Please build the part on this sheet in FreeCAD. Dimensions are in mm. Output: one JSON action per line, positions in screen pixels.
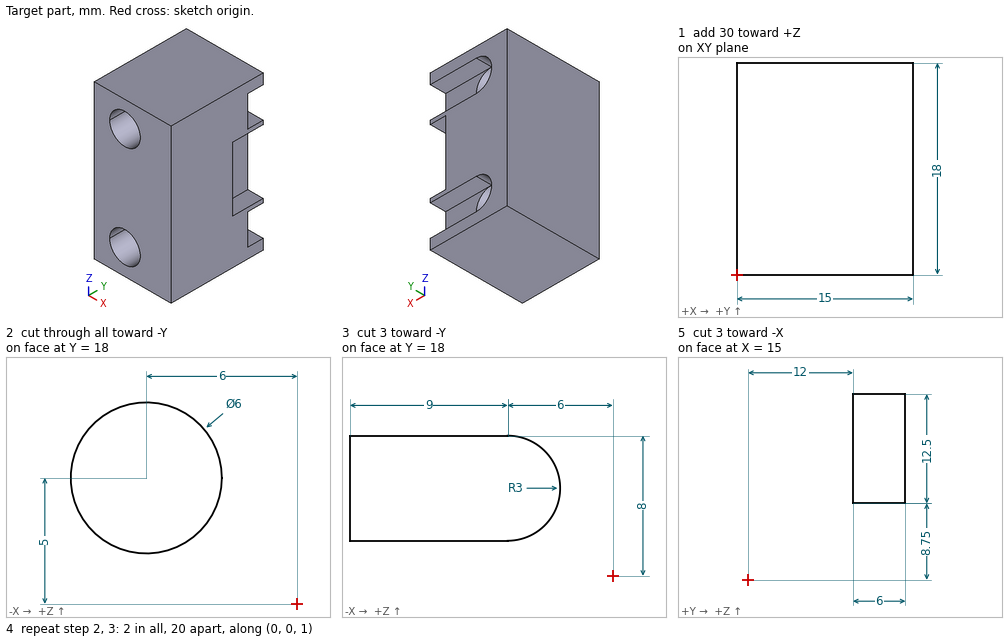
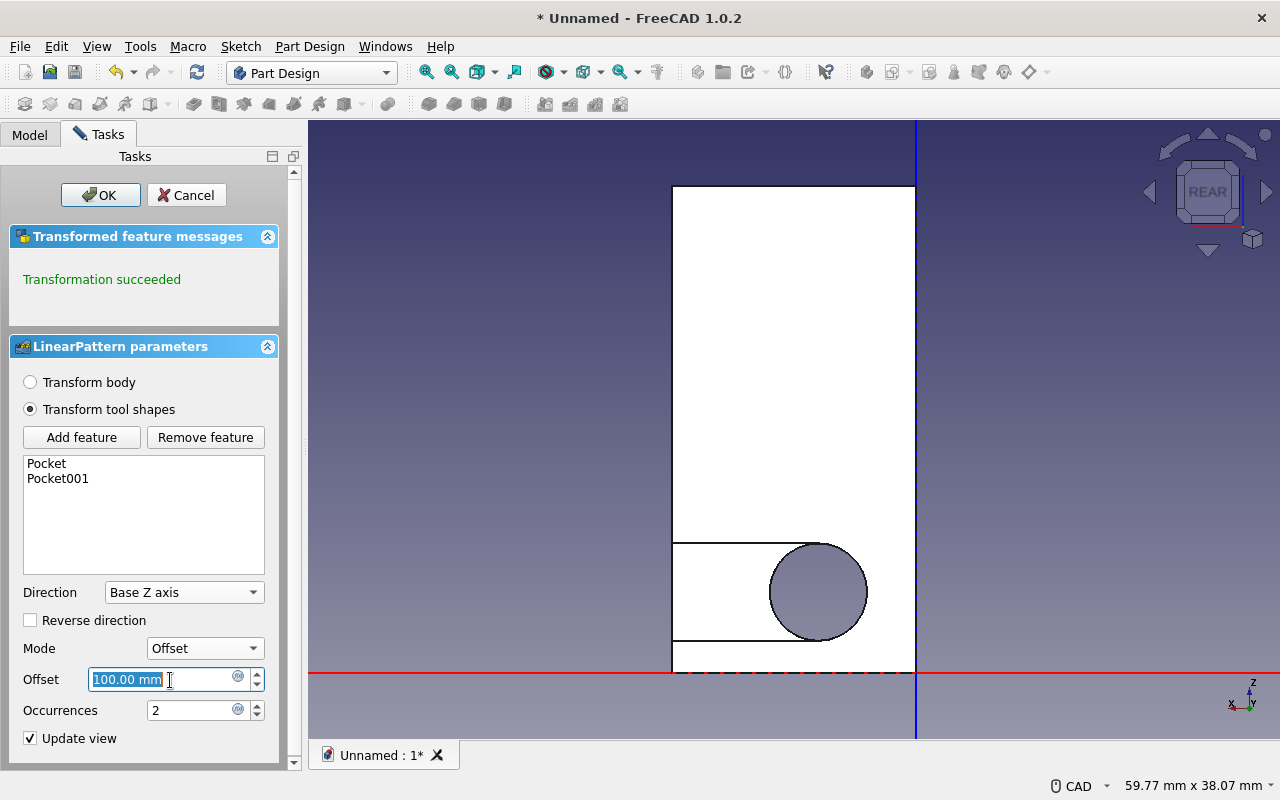
{"action": "type", "text": "20"}
{"action": "key", "text": "Tab"}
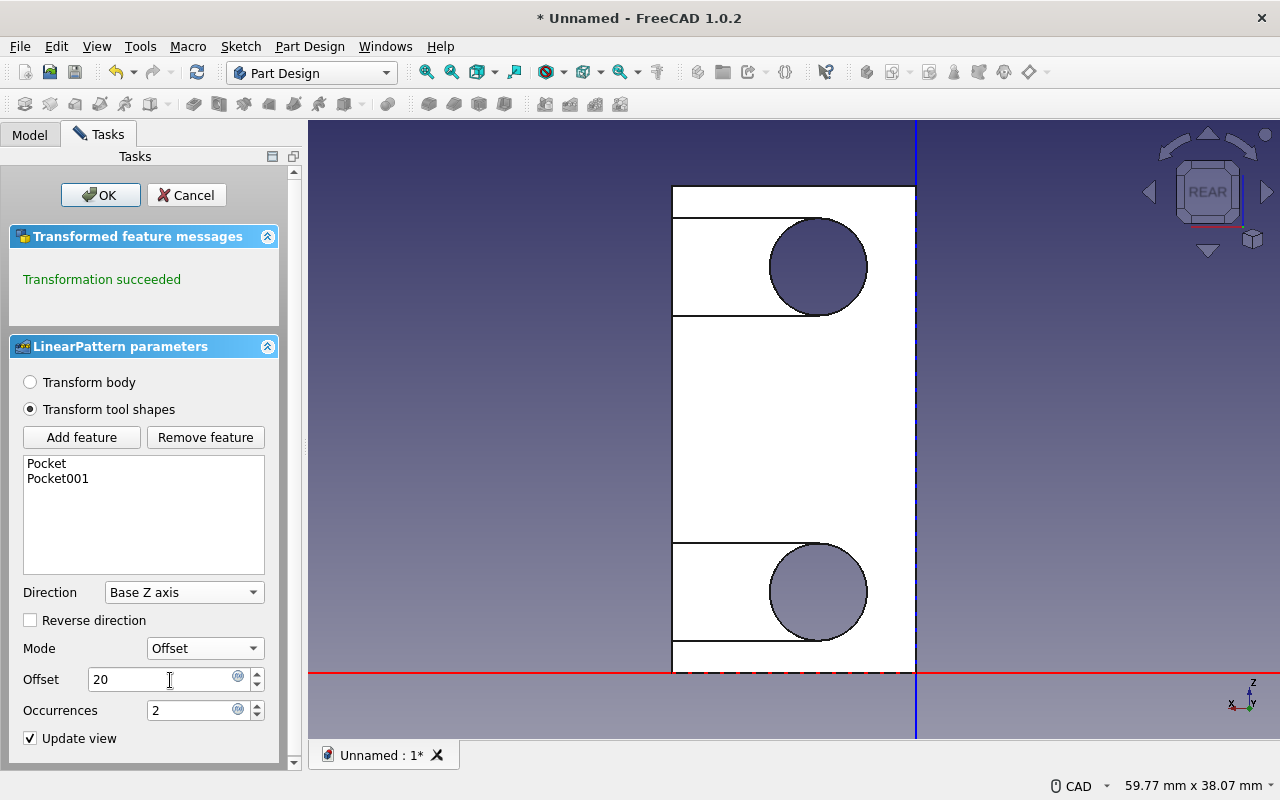
{"action": "triple_click", "coordinate": [199, 710]}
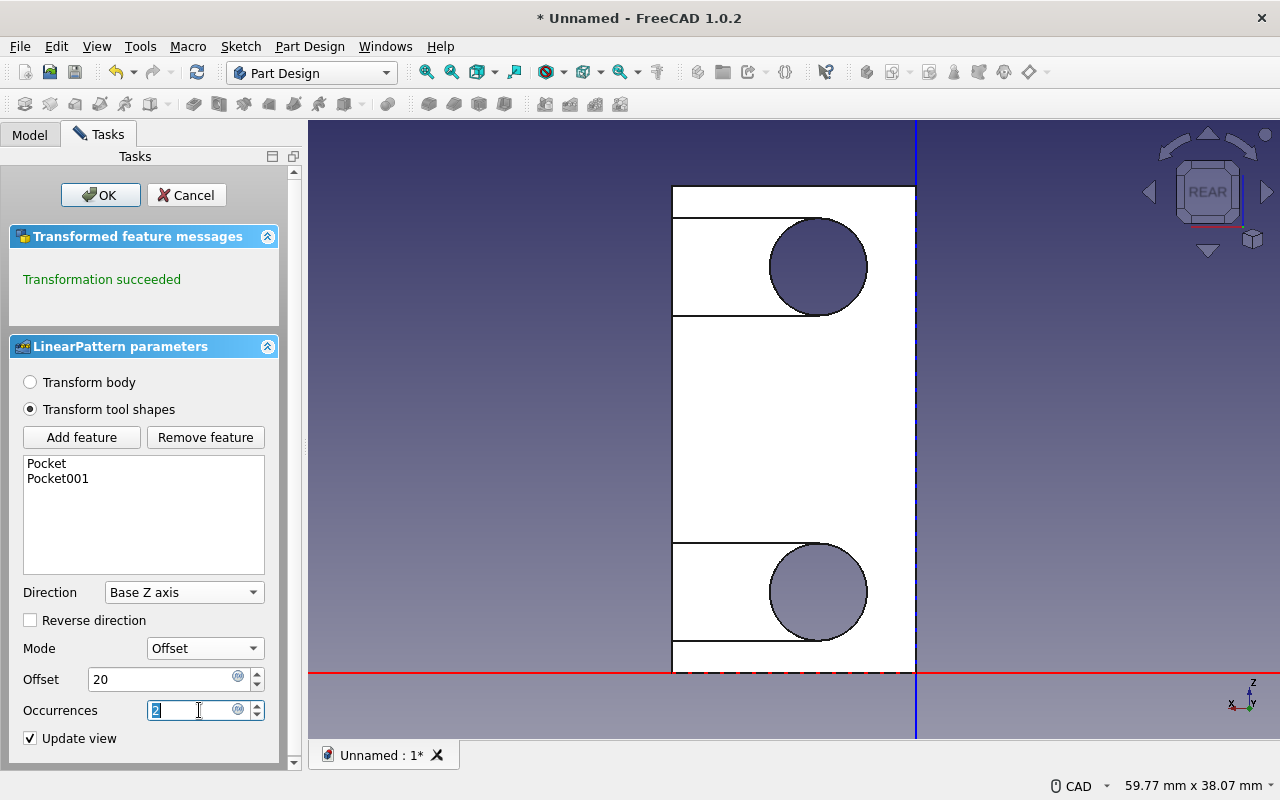
{"action": "type", "text": "2"}
{"action": "key", "text": "Tab"}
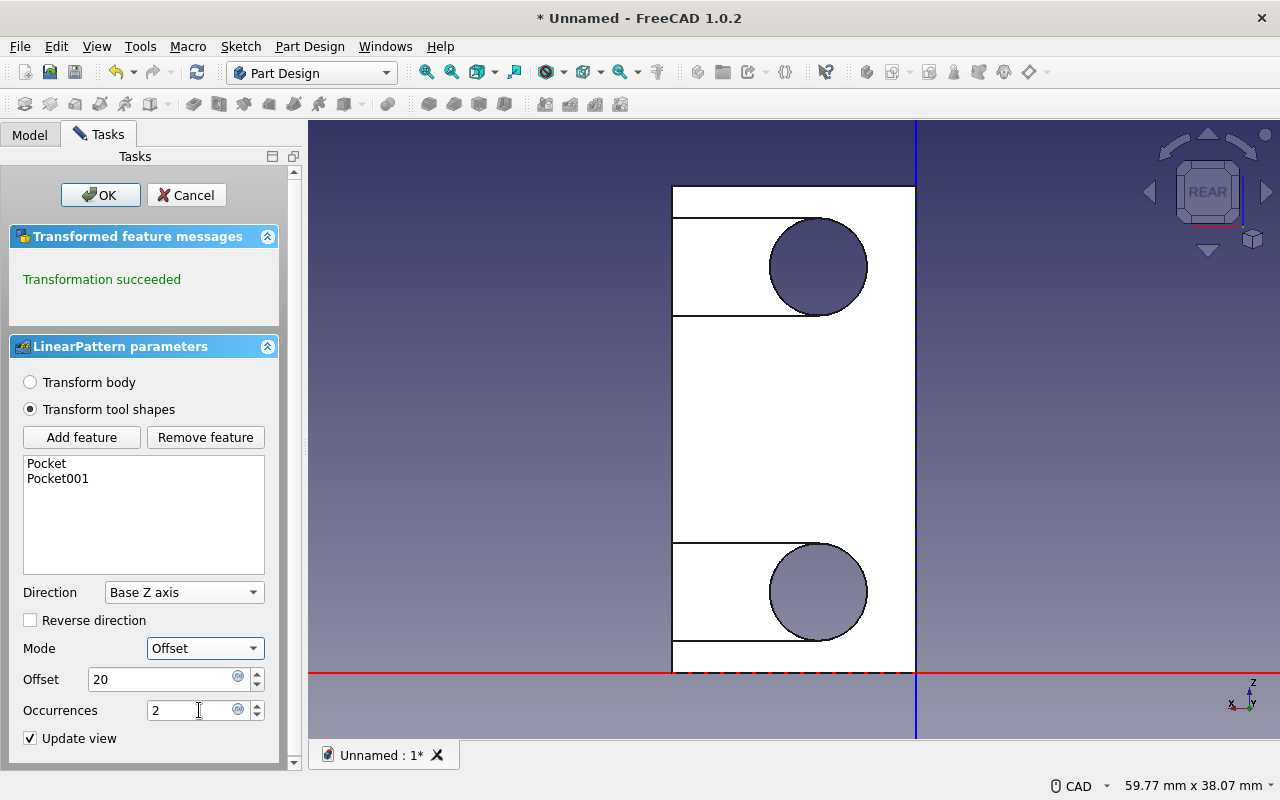
{"action": "left_click", "coordinate": [101, 195]}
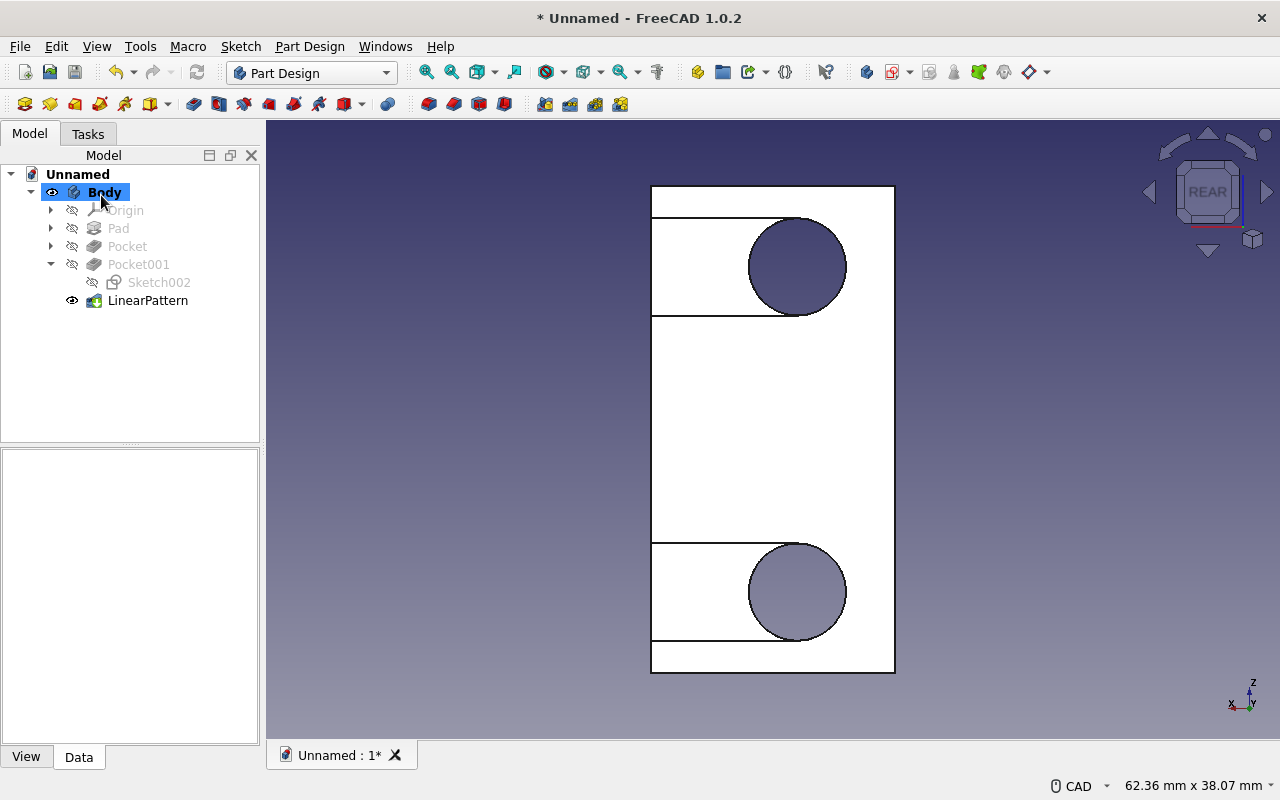
{"action": "key", "text": "0"}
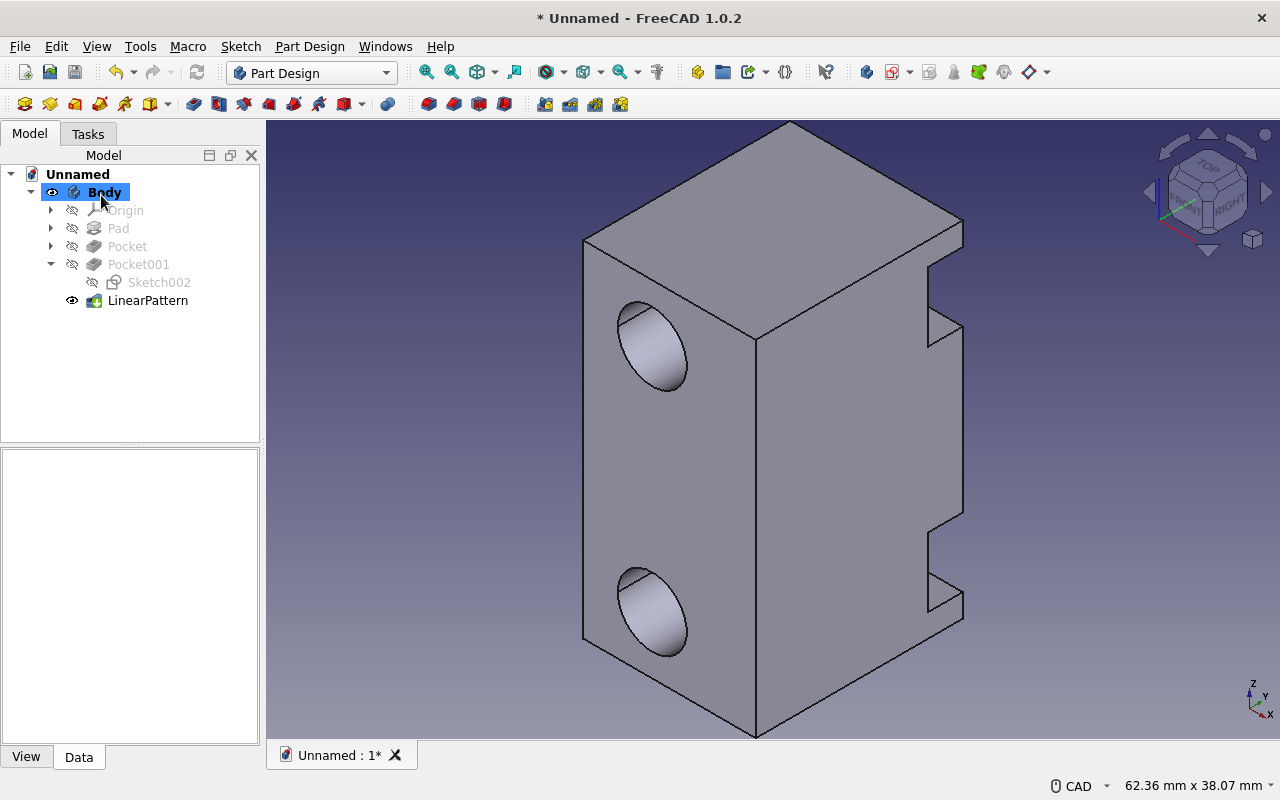
{"action": "left_click", "coordinate": [859, 478]}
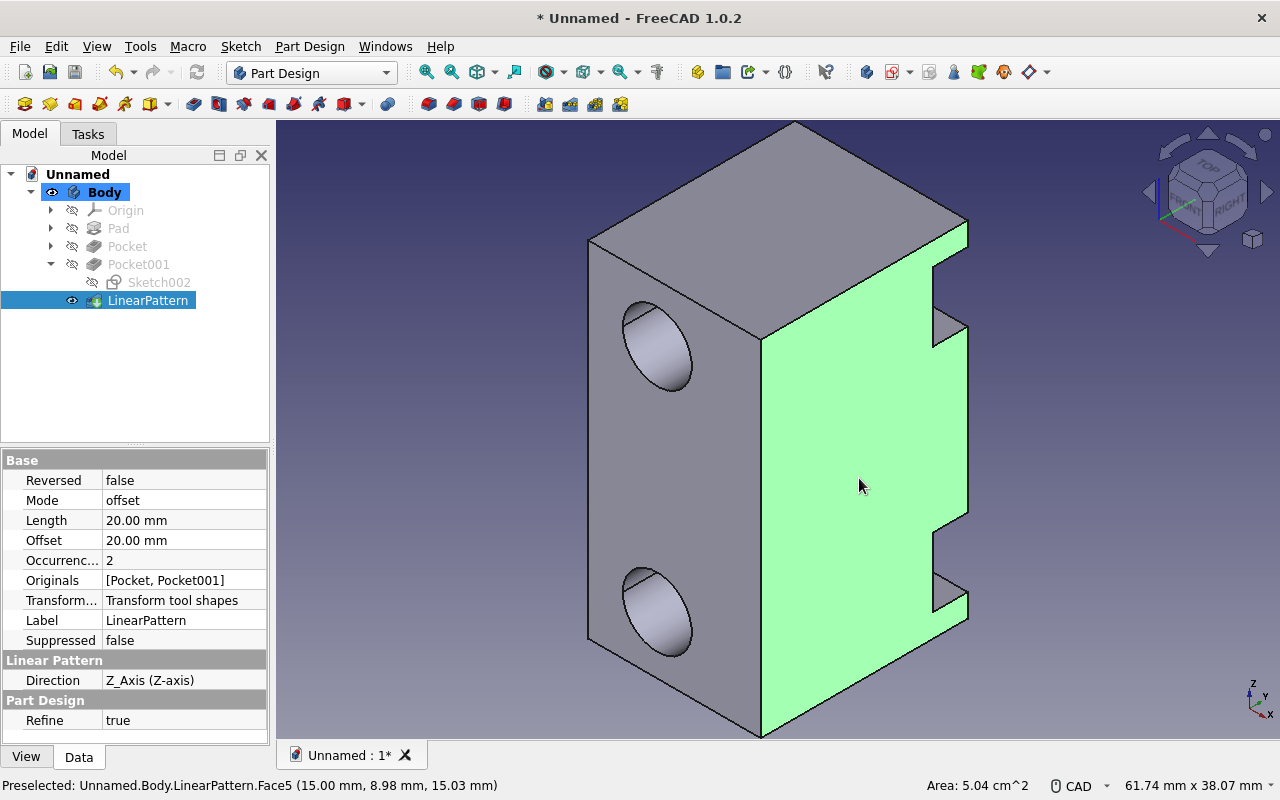
{"action": "left_click", "coordinate": [892, 72]}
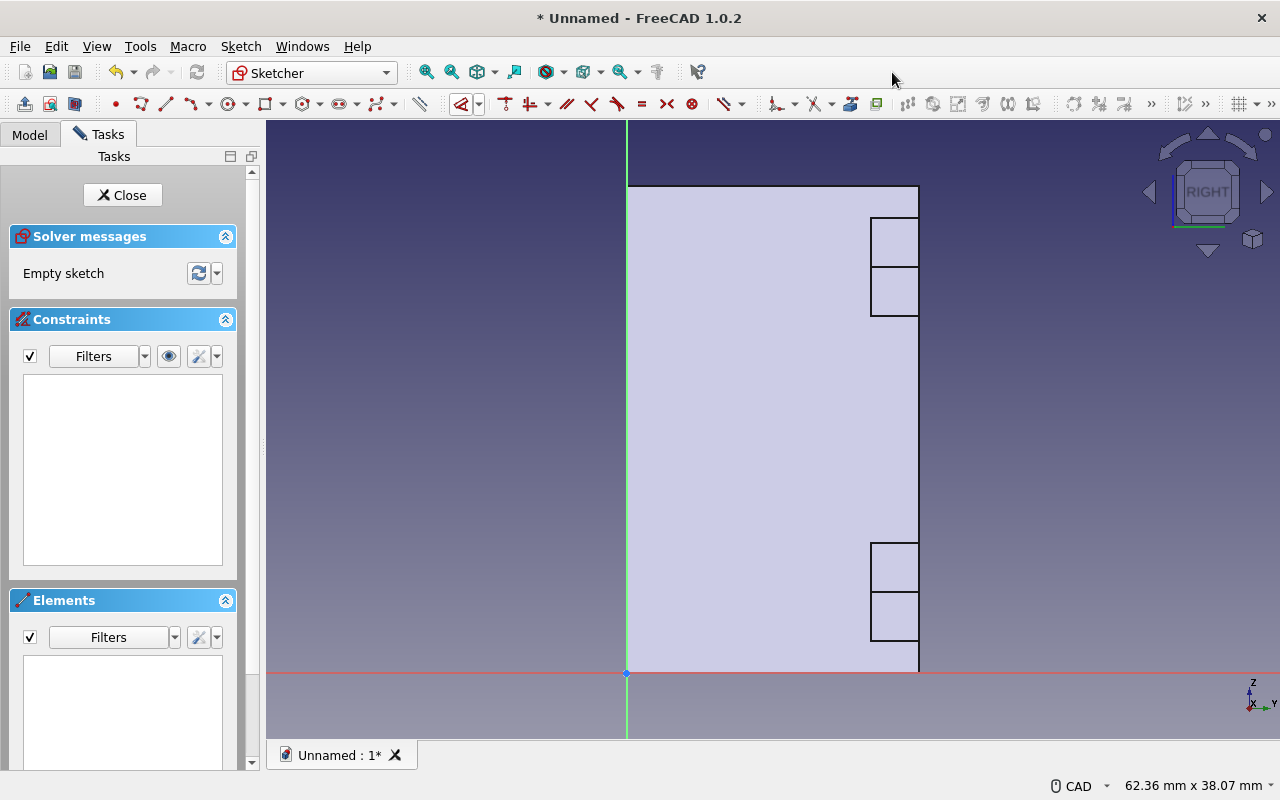
{"action": "left_click", "coordinate": [264, 104]}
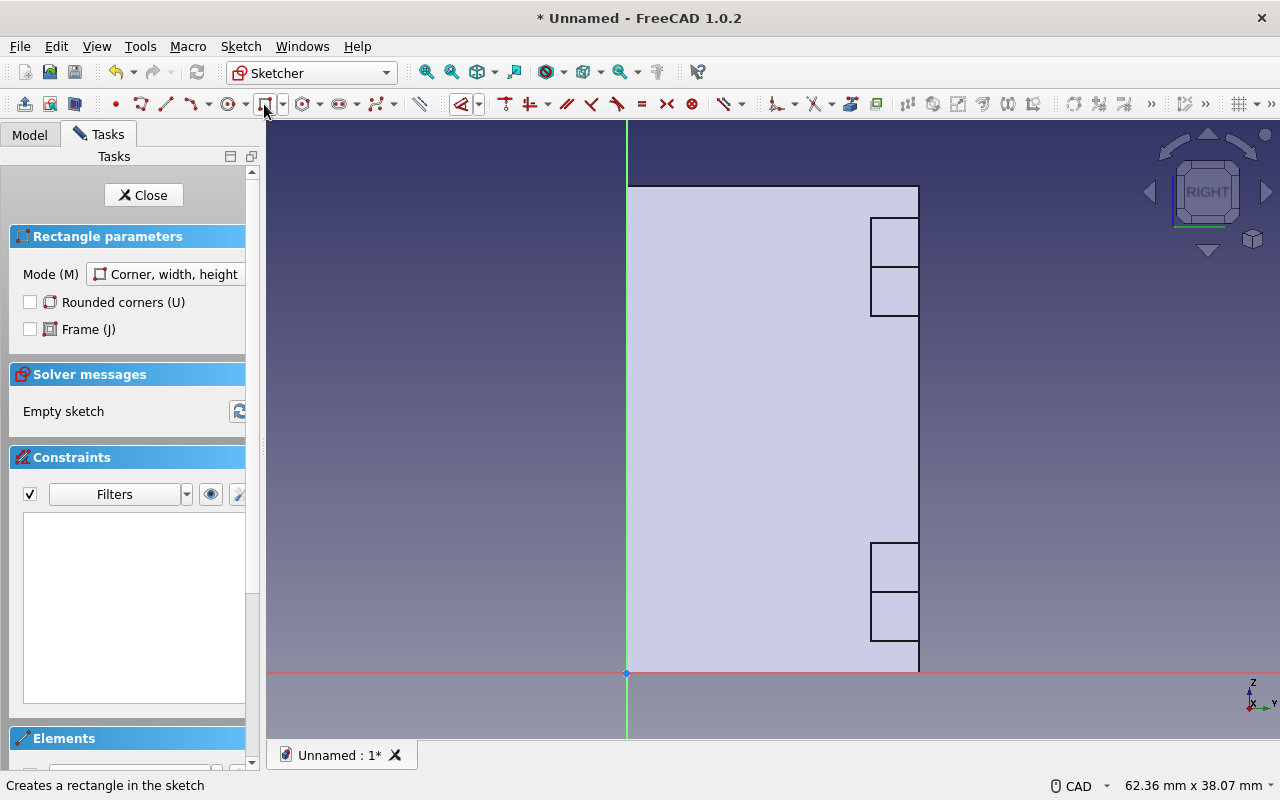
{"action": "left_click", "coordinate": [822, 328]}
{"action": "mouse_move", "coordinate": [919, 531]}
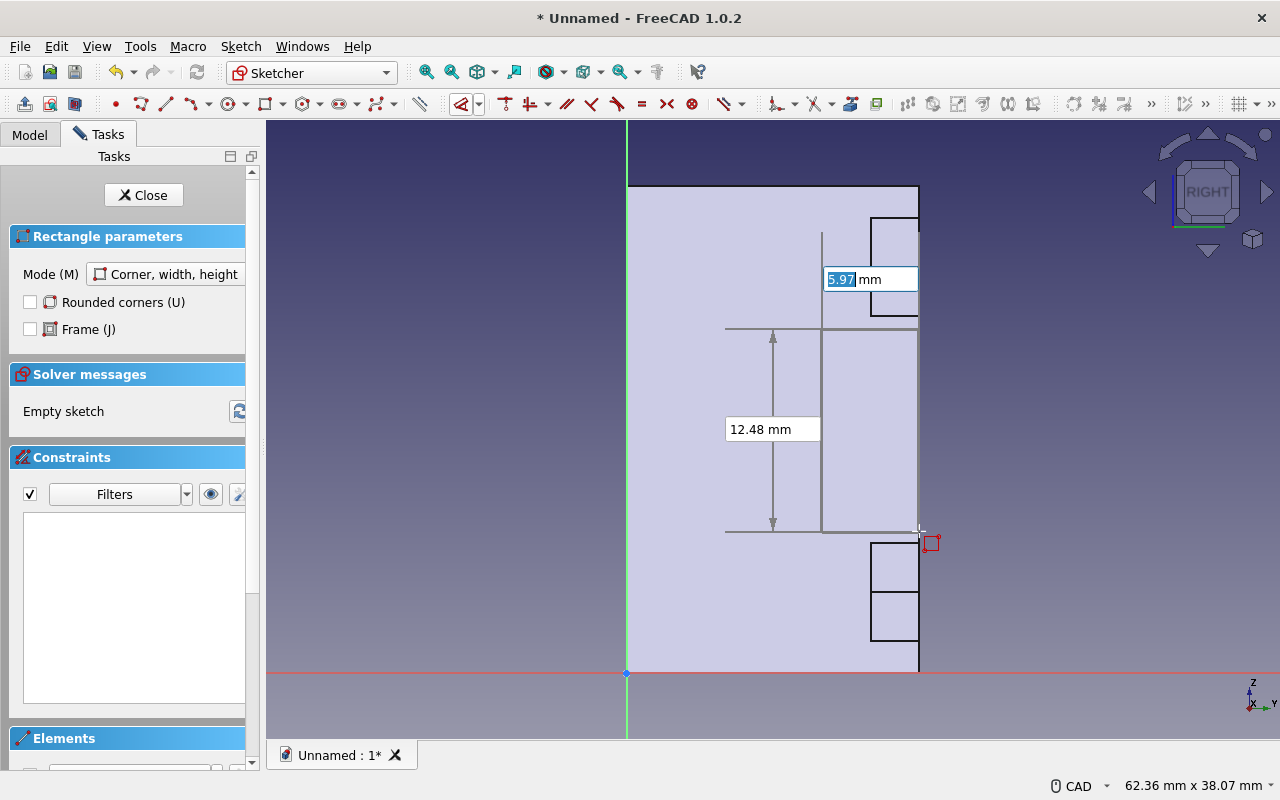
{"action": "type", "text": "6"}
{"action": "key", "text": "Tab"}
{"action": "type", "text": "12.5"}
{"action": "key", "text": "Return"}
{"action": "key", "text": "Escape"}